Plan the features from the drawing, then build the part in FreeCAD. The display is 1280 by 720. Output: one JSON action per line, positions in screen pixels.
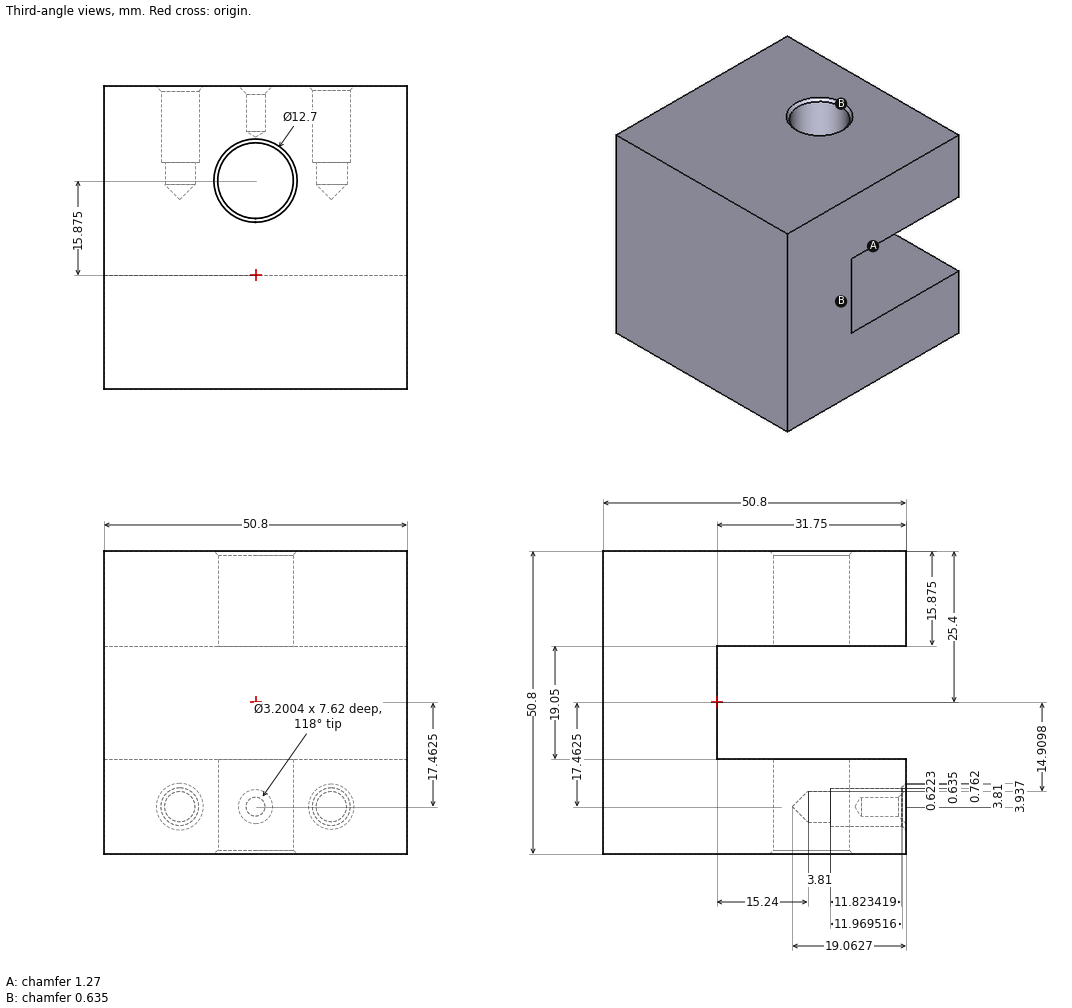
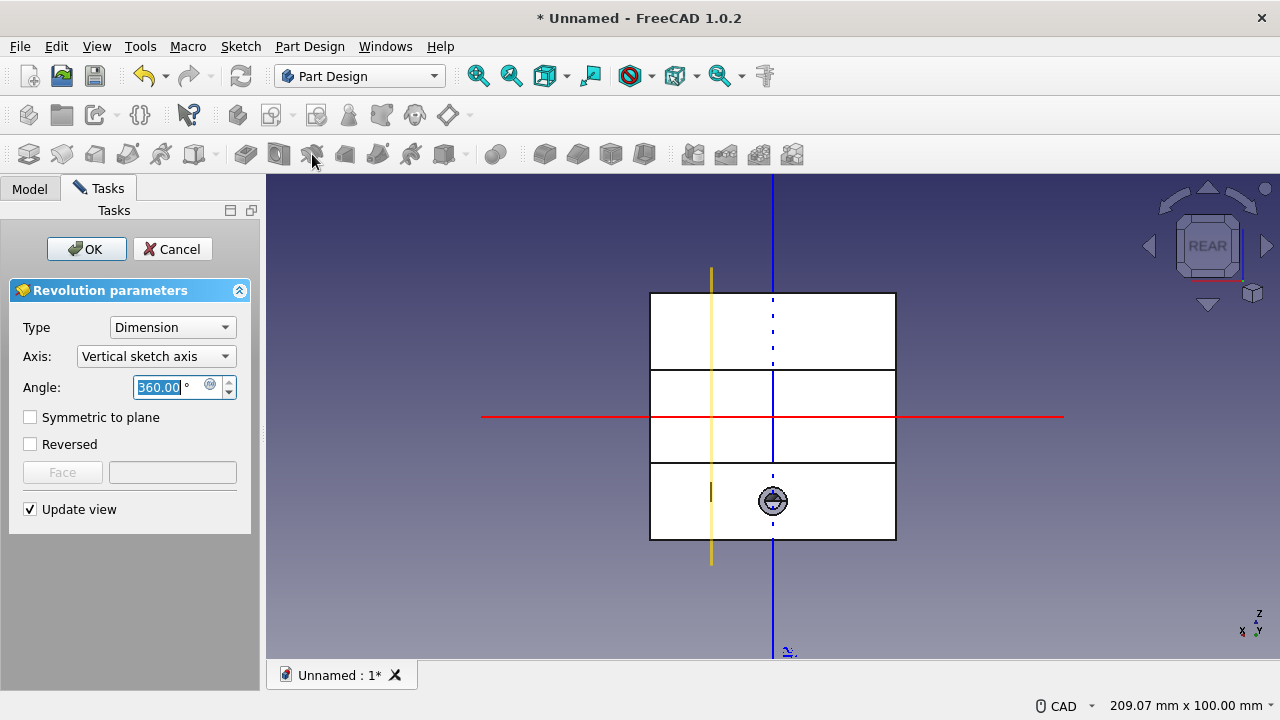
{"action": "left_click", "coordinate": [157, 356]}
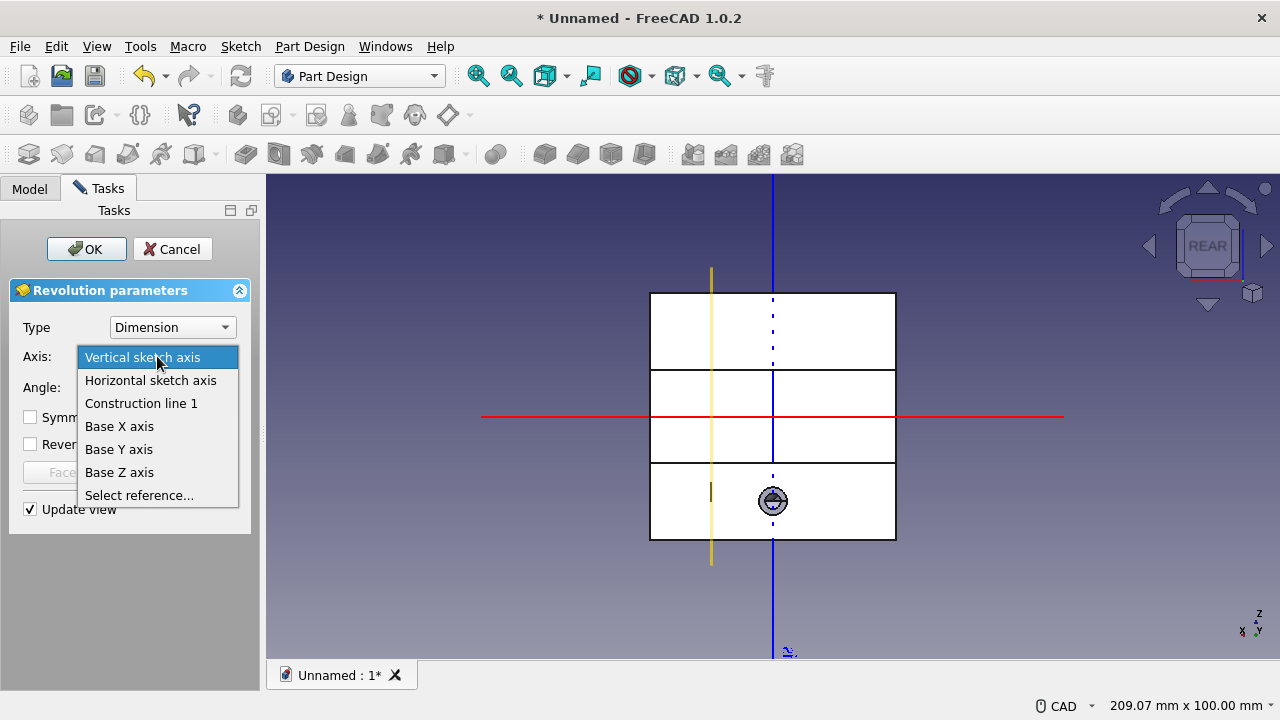
{"action": "left_click", "coordinate": [156, 404]}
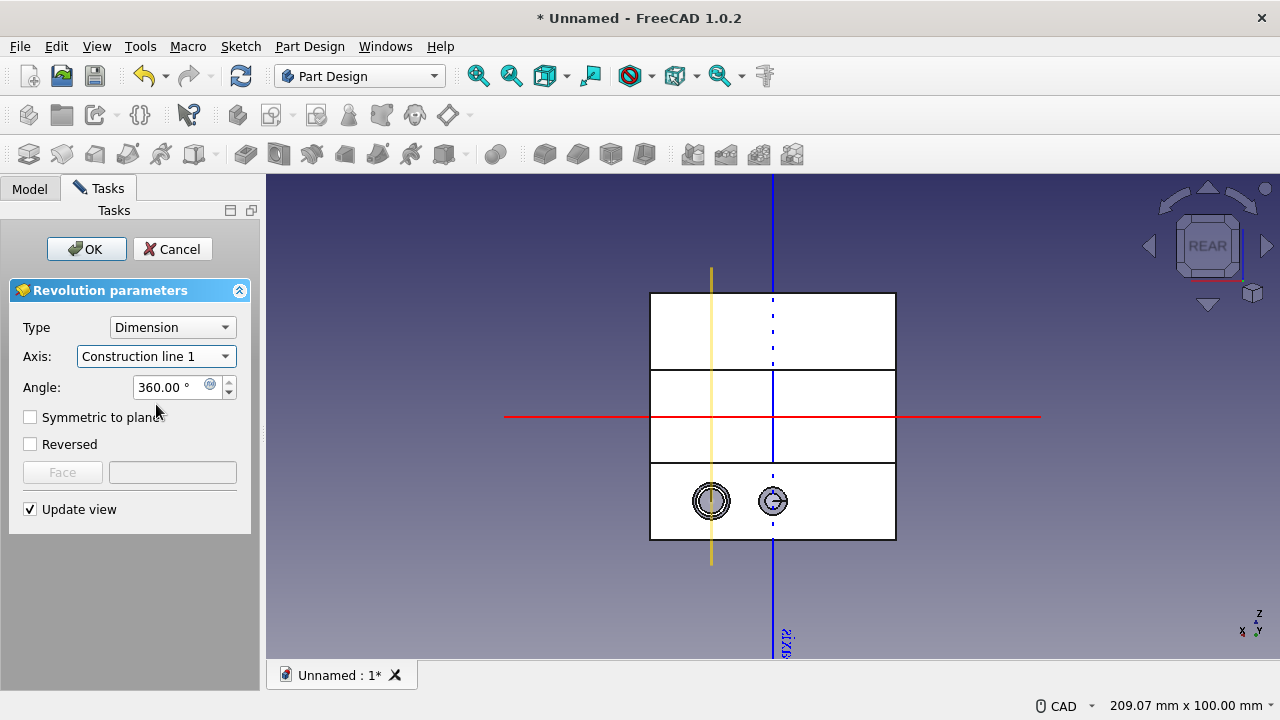
{"action": "left_click", "coordinate": [87, 249]}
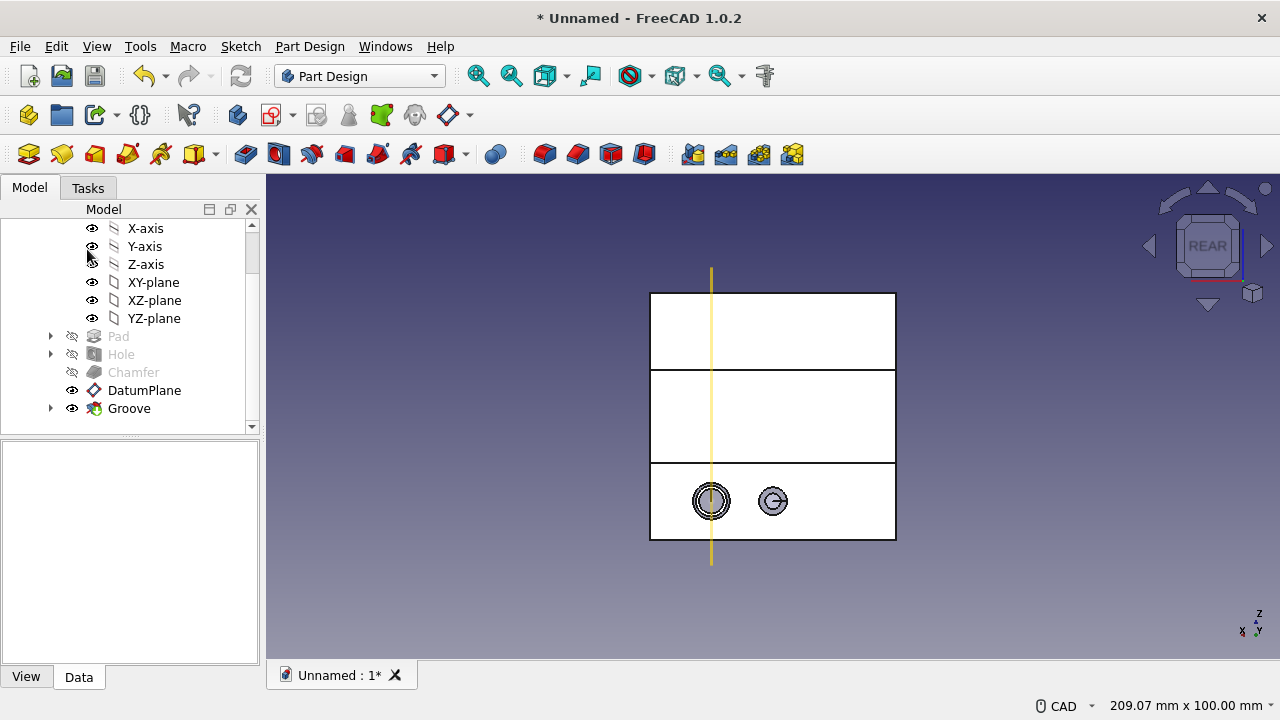
{"action": "left_click", "coordinate": [117, 390]}
{"action": "key", "text": "space"}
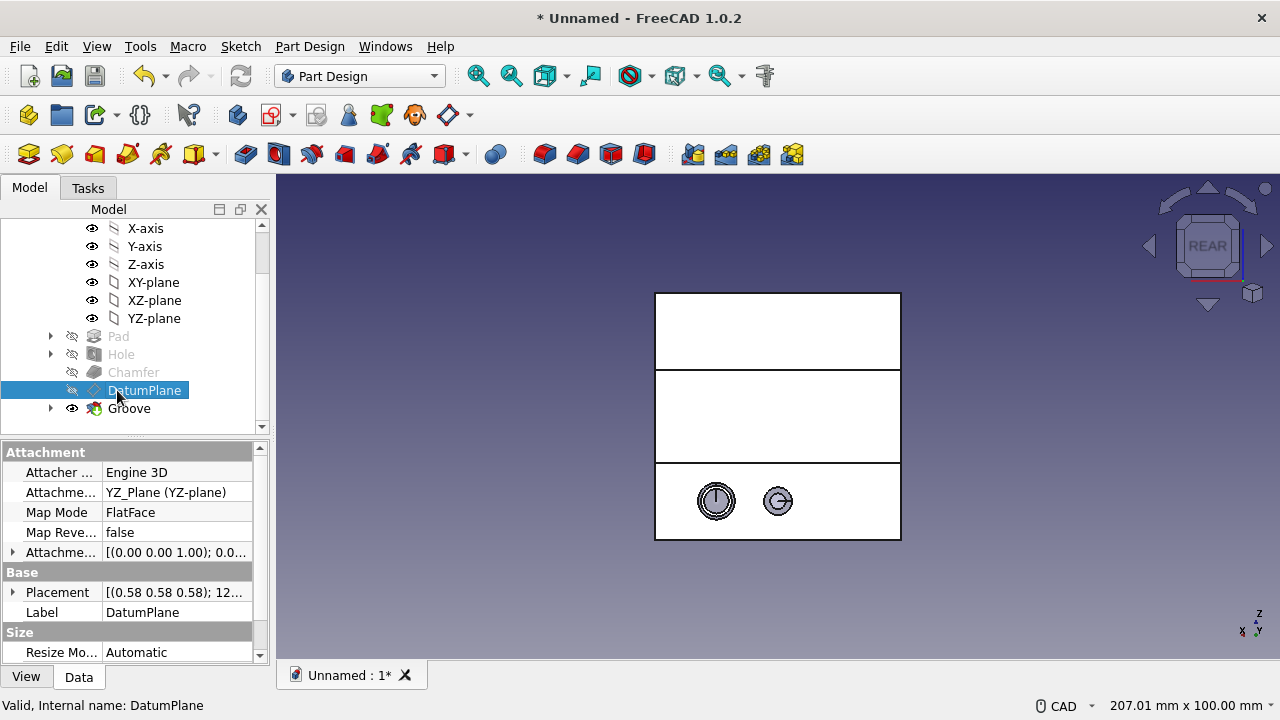
{"action": "scroll", "coordinate": [161, 314], "scroll_direction": "down", "scroll_amount": 3}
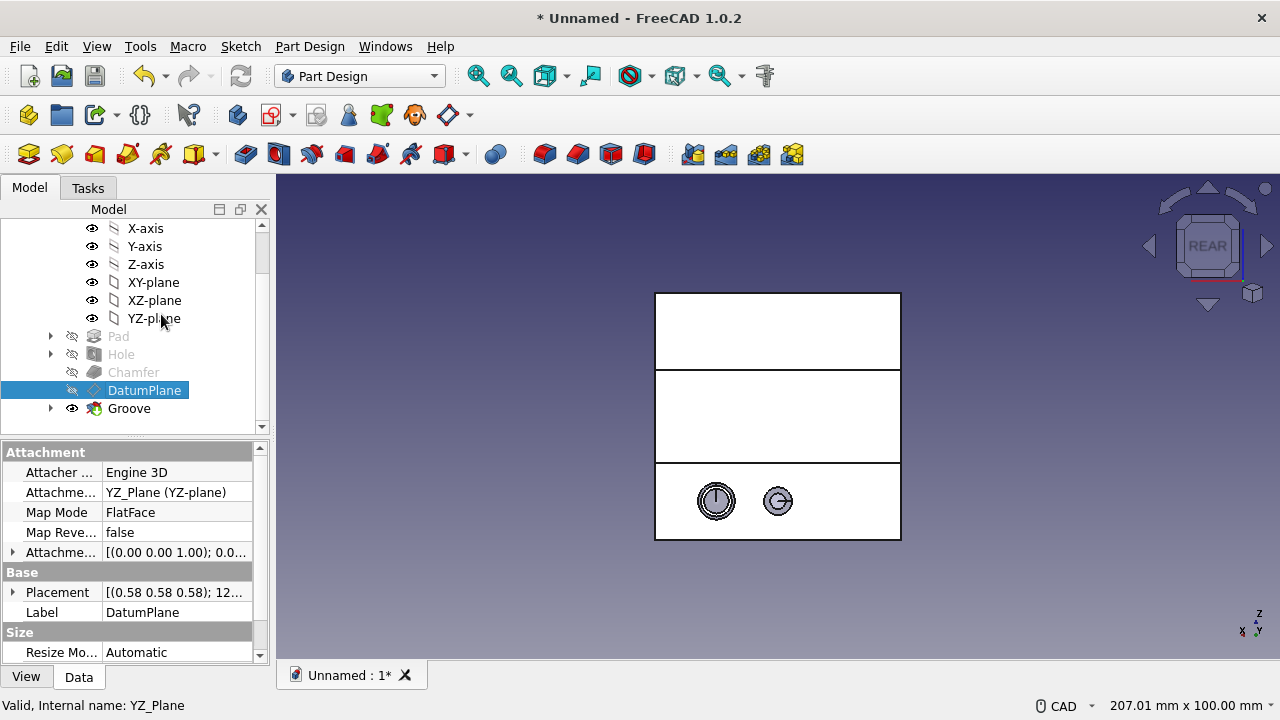
{"action": "scroll", "coordinate": [161, 314], "scroll_direction": "up", "scroll_amount": 15}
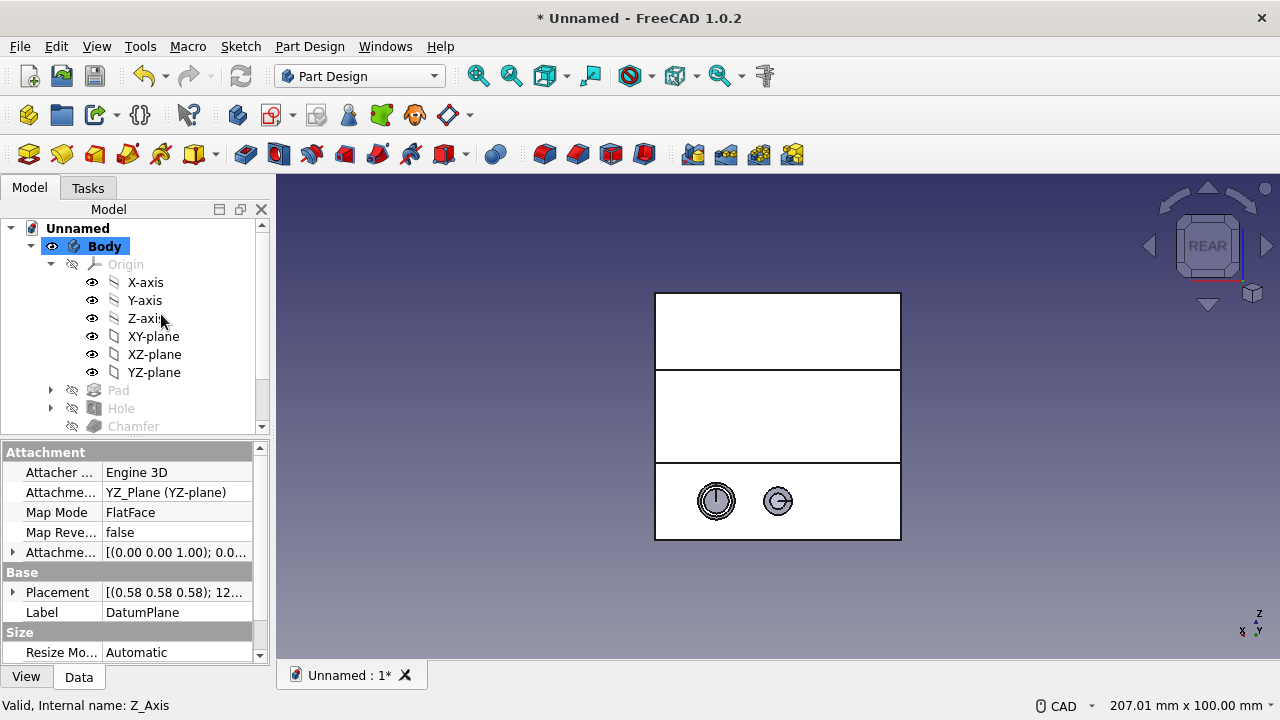
{"action": "left_click", "coordinate": [137, 372]}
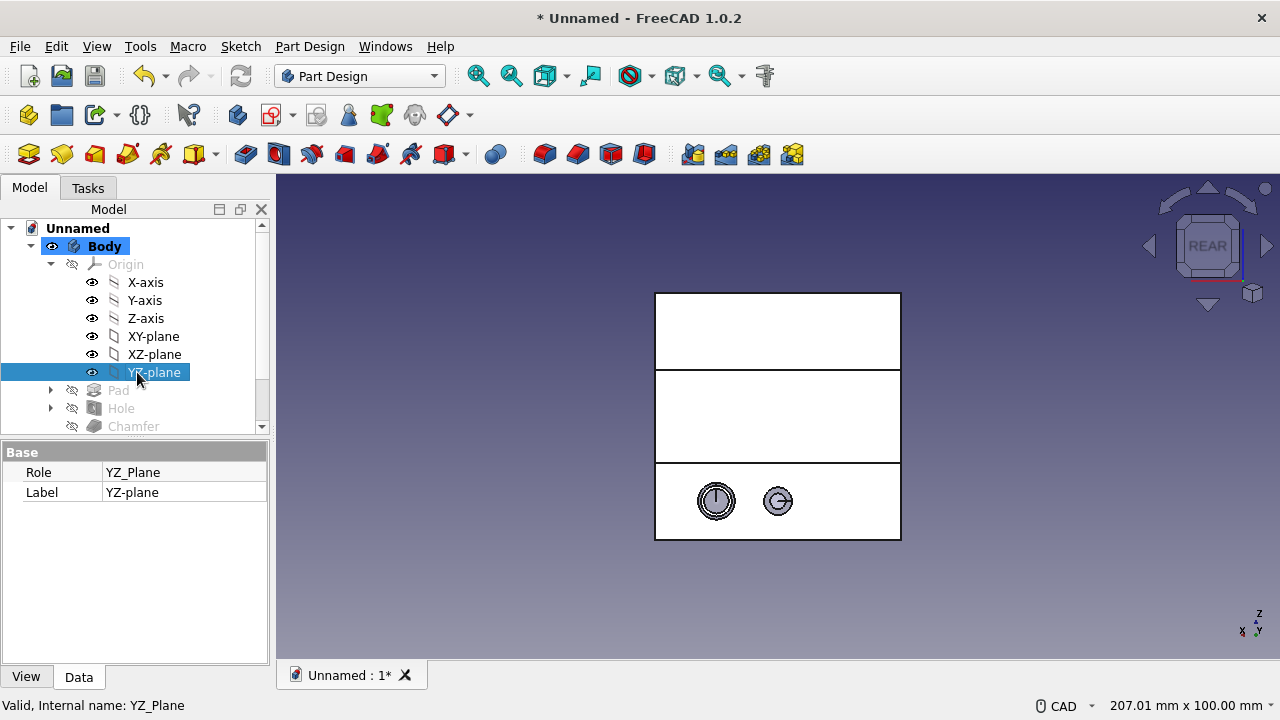
{"action": "left_click", "coordinate": [448, 116]}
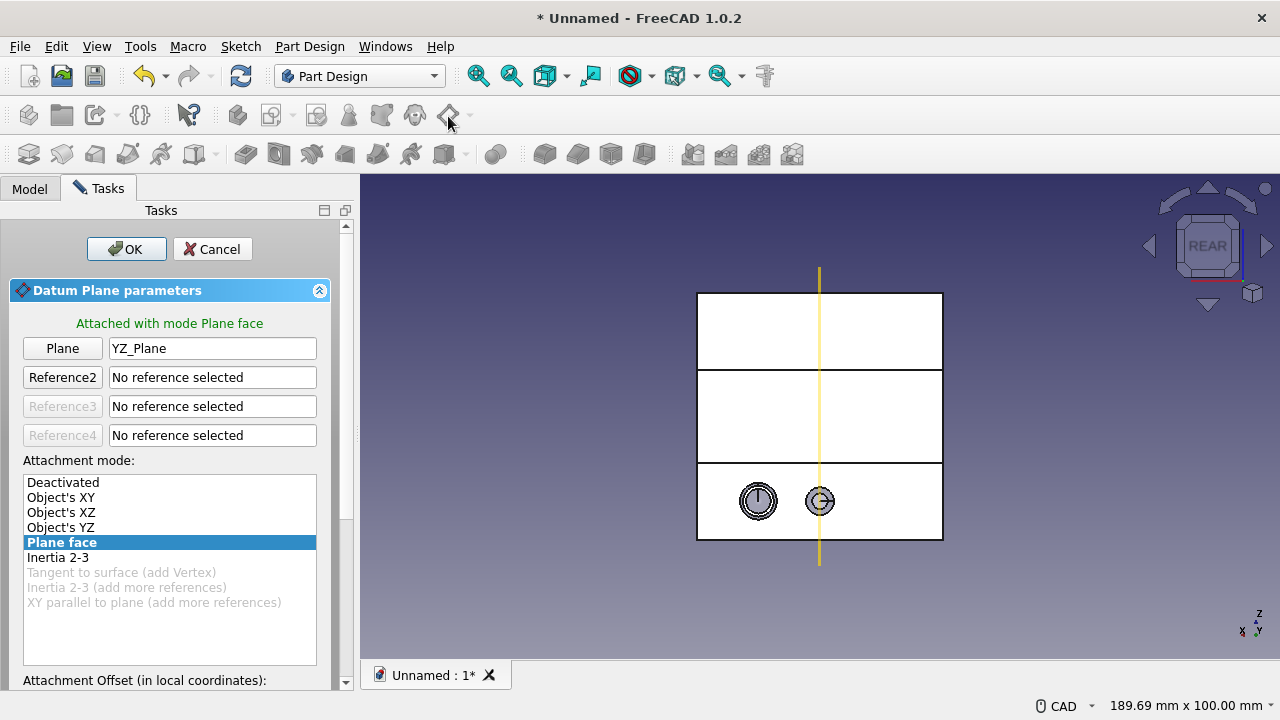
{"action": "scroll", "coordinate": [346, 455], "scroll_direction": "down", "scroll_amount": 3}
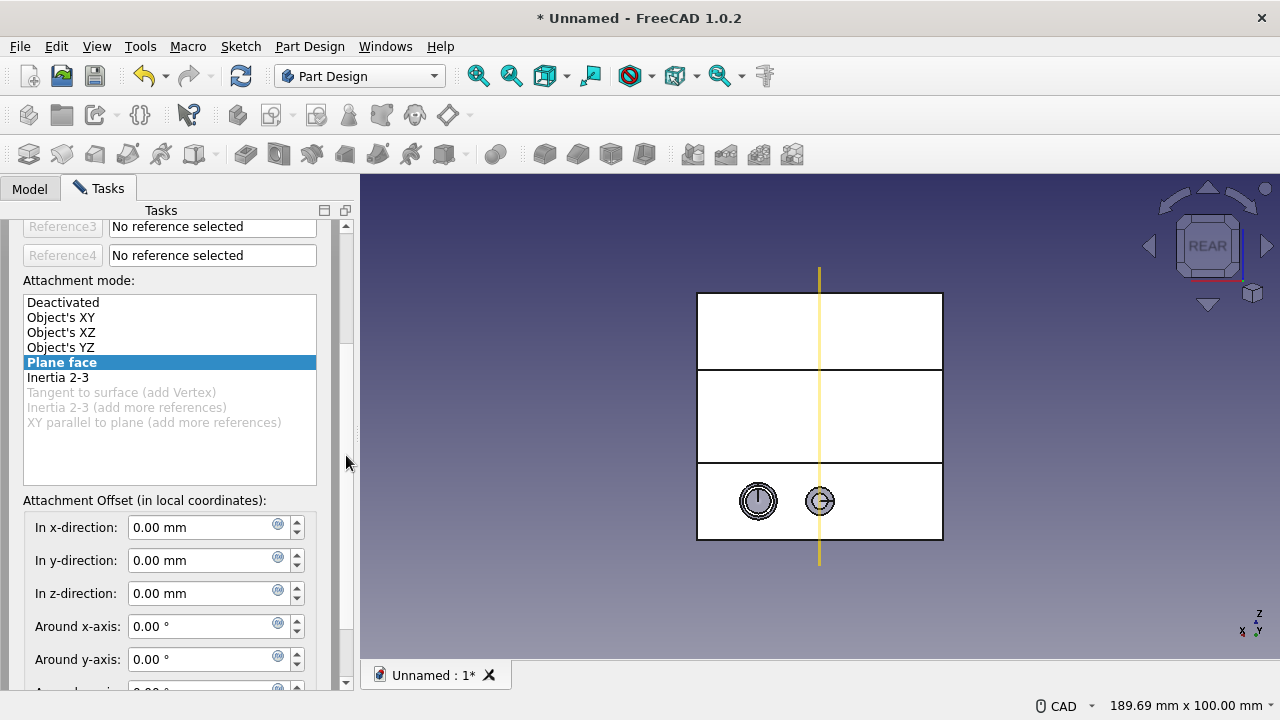
{"action": "triple_click", "coordinate": [210, 594]}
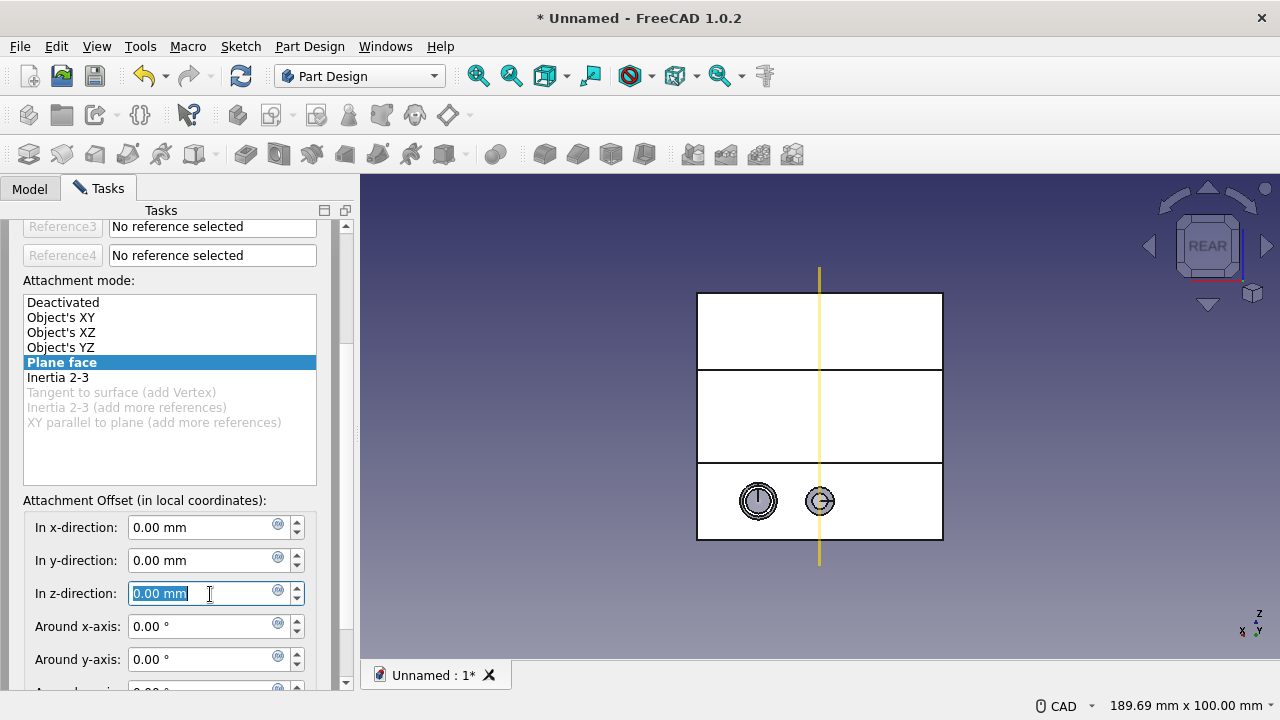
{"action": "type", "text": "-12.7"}
{"action": "key", "text": "Tab"}